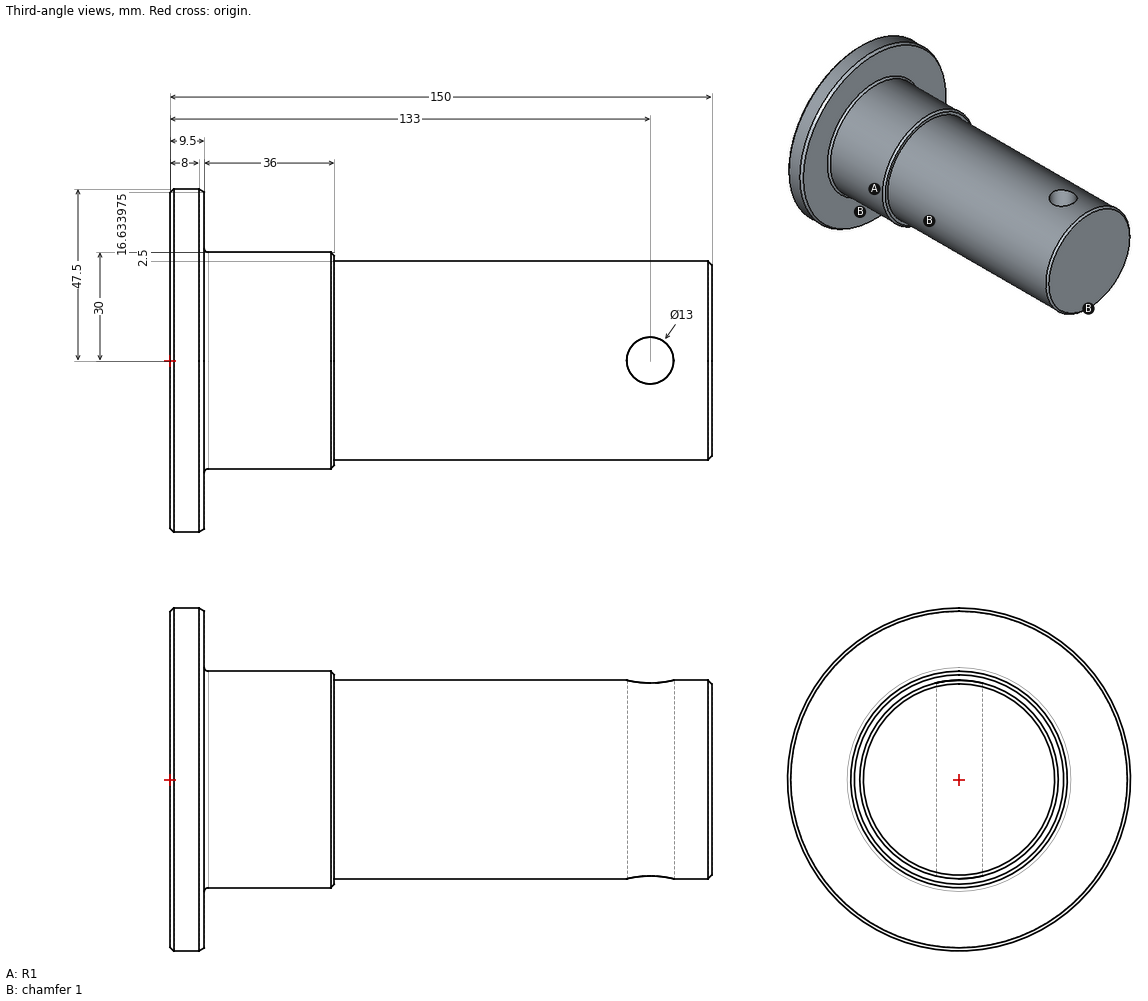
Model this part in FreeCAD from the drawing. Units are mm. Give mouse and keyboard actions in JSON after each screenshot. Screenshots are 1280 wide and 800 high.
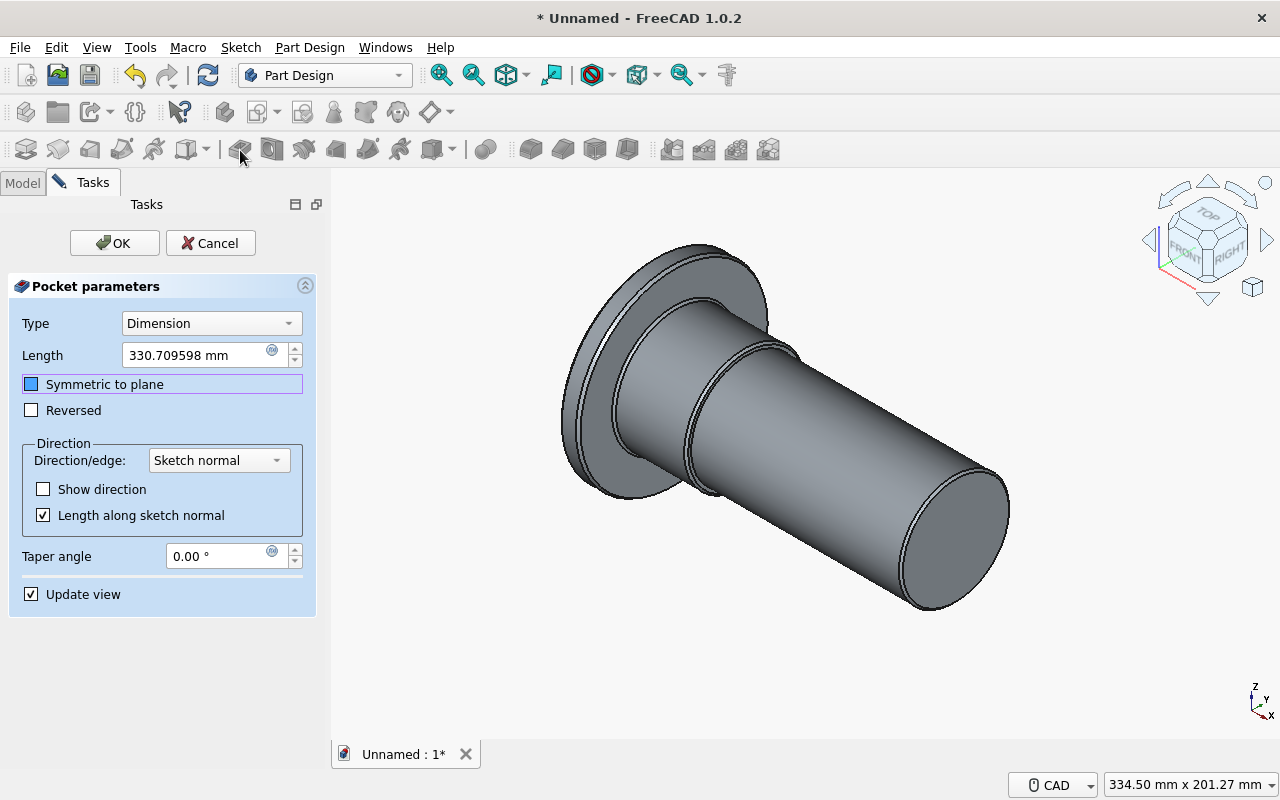
{"action": "left_click", "coordinate": [30, 384]}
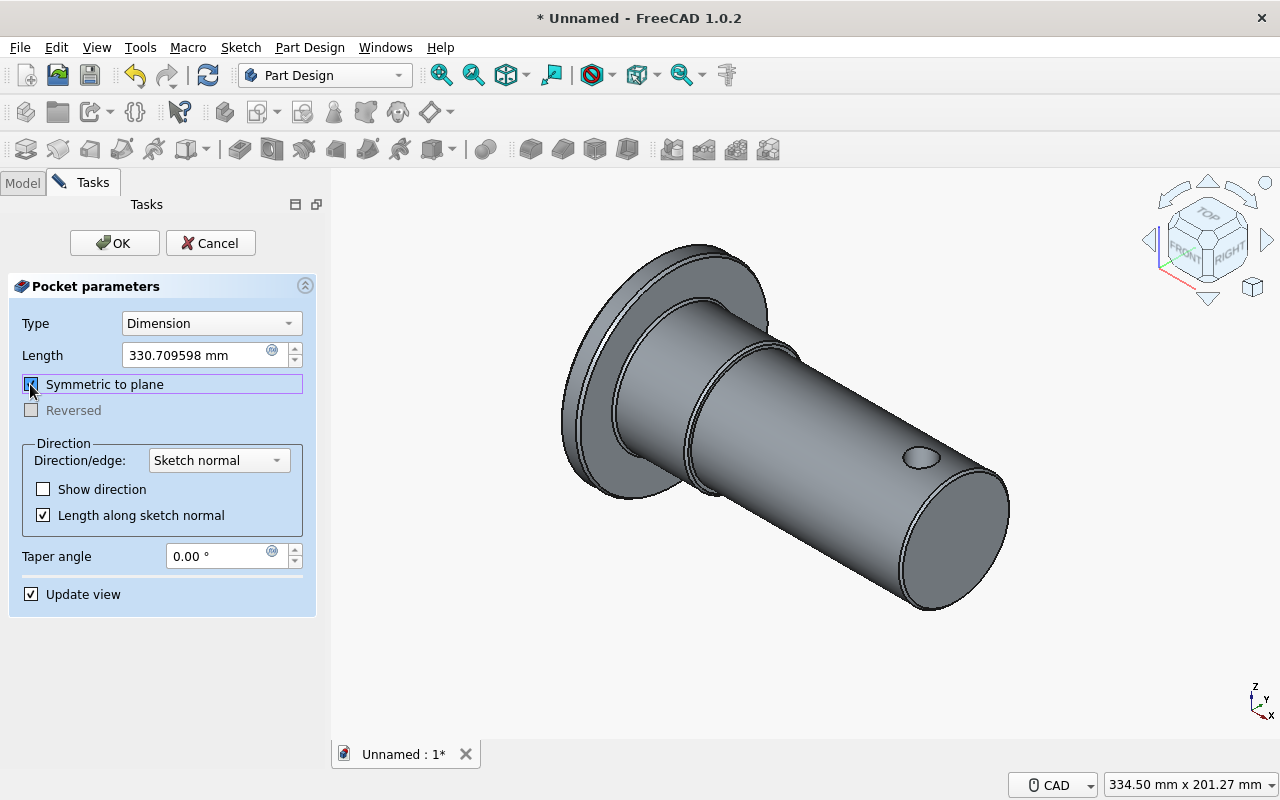
{"action": "left_click", "coordinate": [115, 243]}